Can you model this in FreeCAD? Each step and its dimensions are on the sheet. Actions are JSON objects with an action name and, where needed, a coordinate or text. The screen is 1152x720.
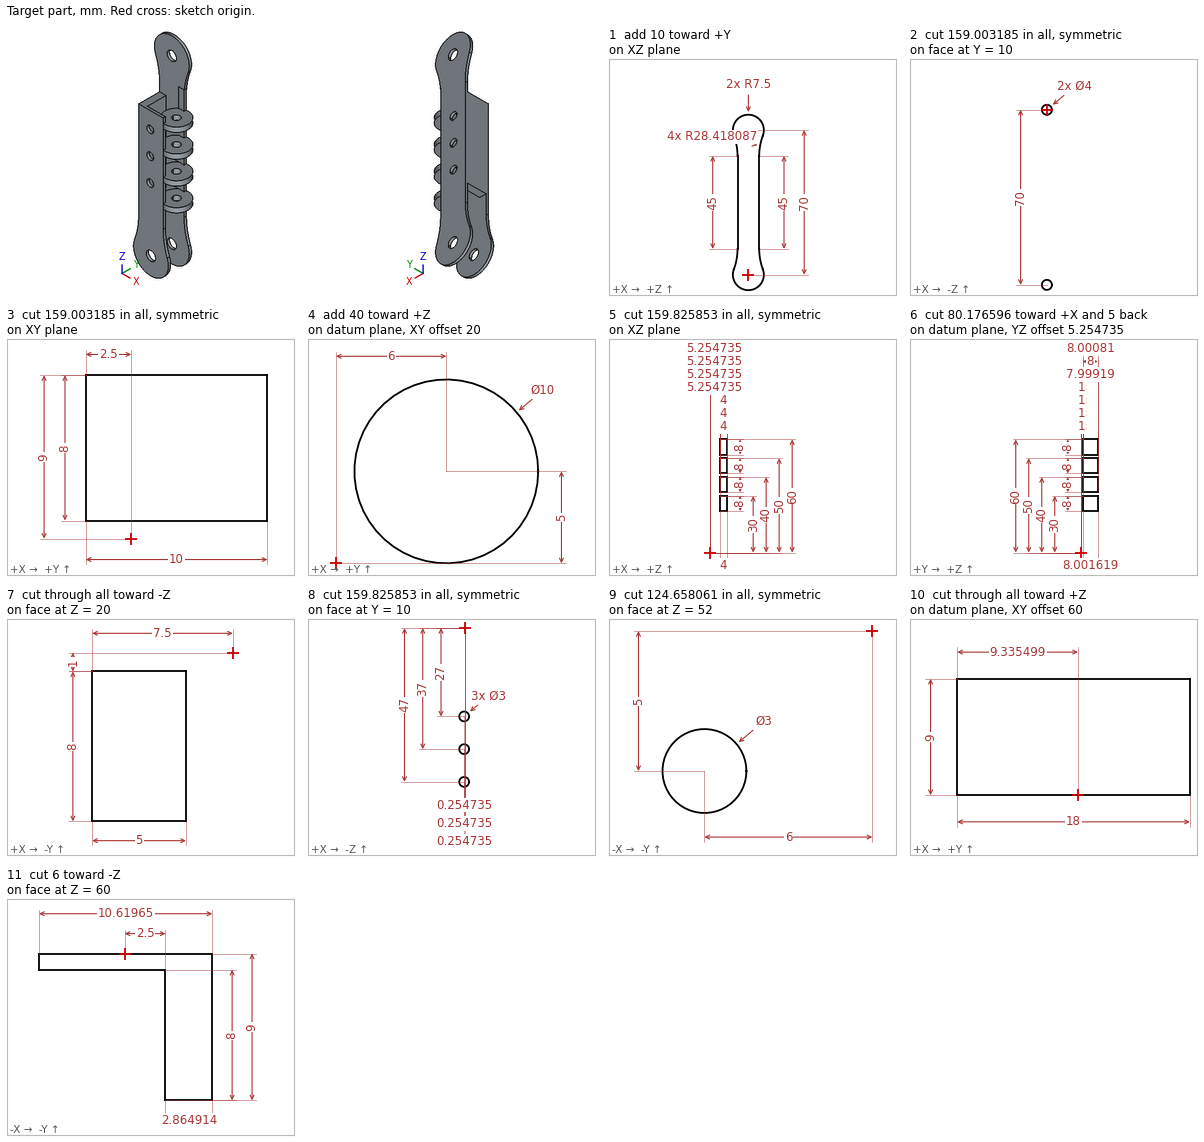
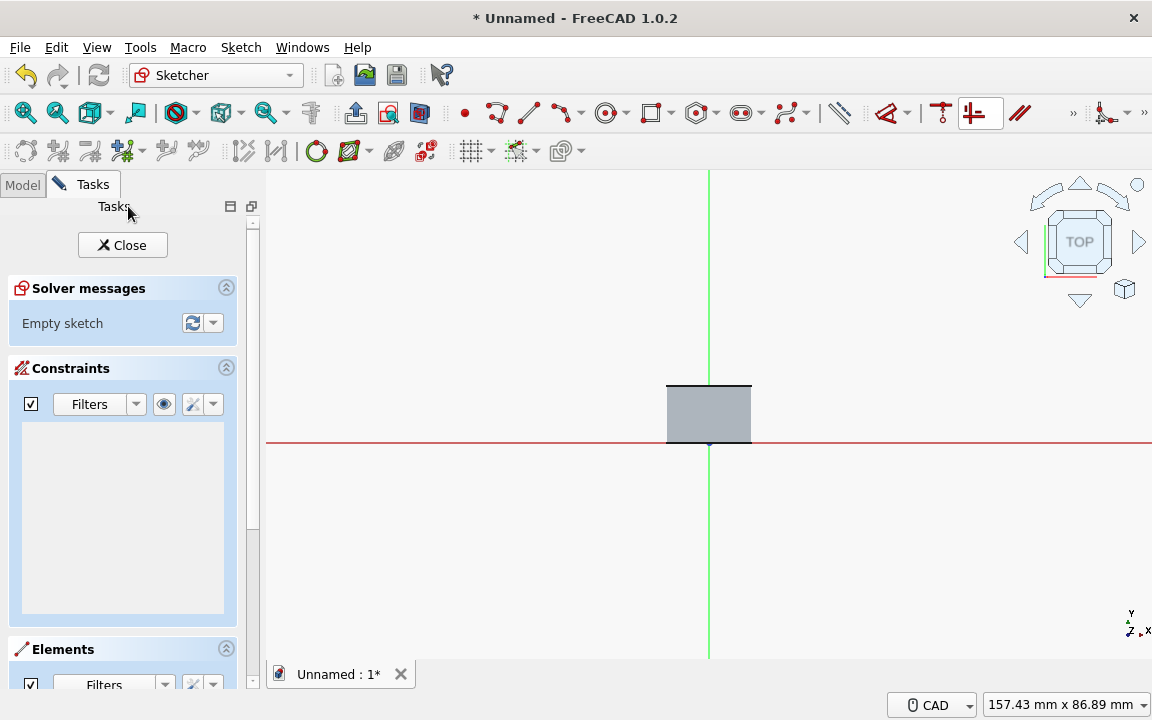
{"action": "left_click", "coordinate": [420, 114]}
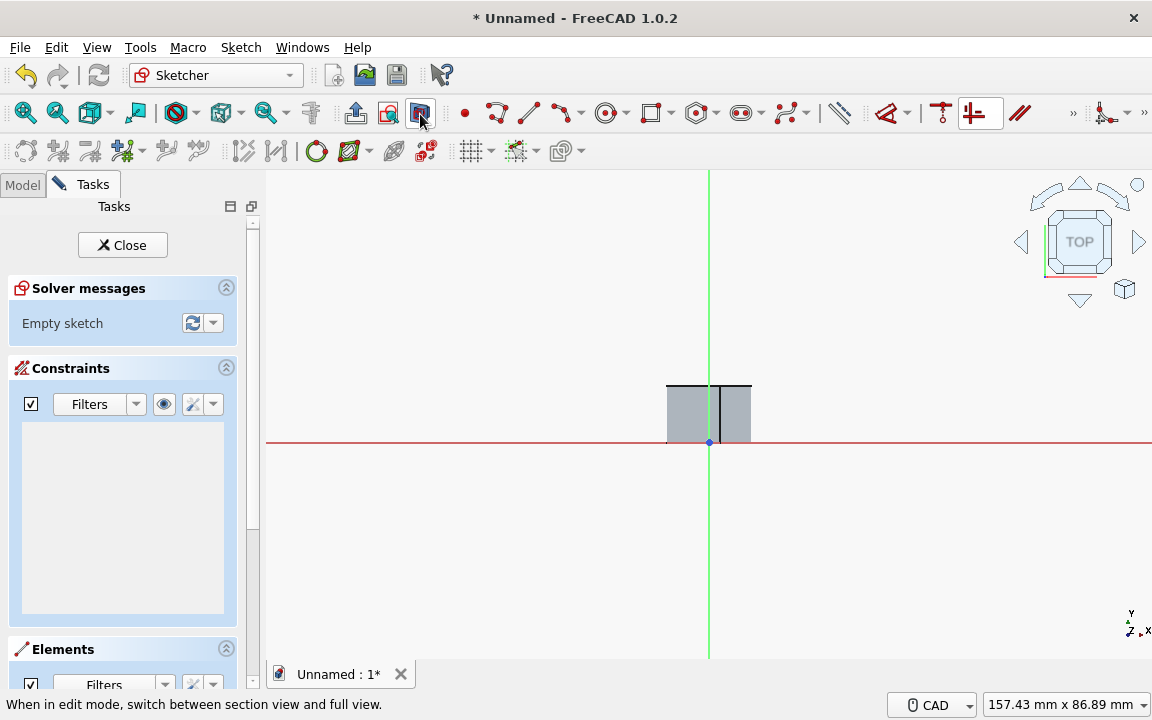
{"action": "scroll", "coordinate": [739, 418], "scroll_direction": "up", "scroll_amount": 9}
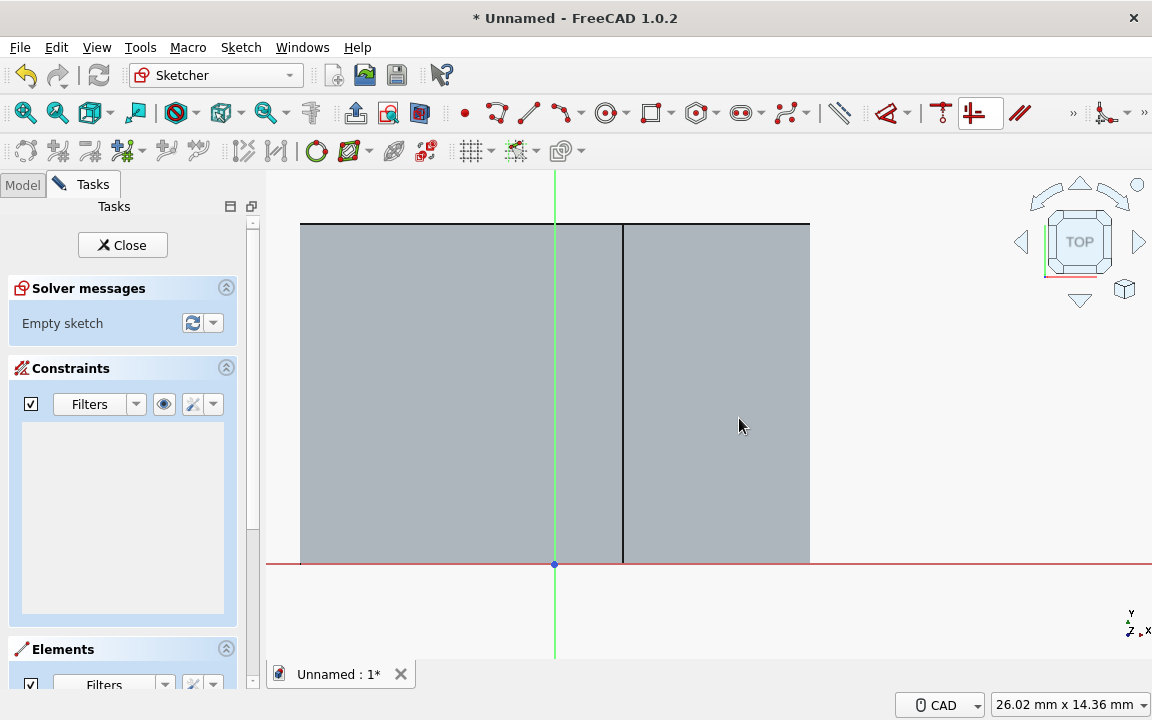
{"action": "left_click", "coordinate": [652, 114]}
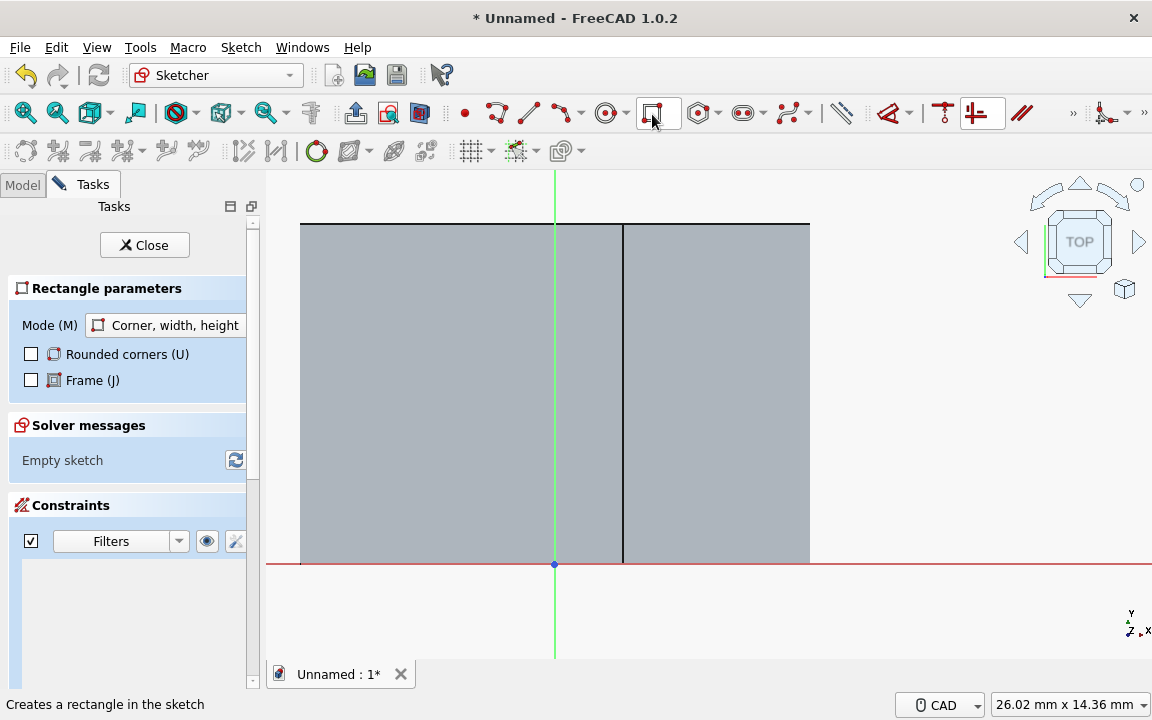
{"action": "left_click", "coordinate": [470, 258]}
{"action": "left_click", "coordinate": [810, 530]}
{"action": "key", "text": "Escape"}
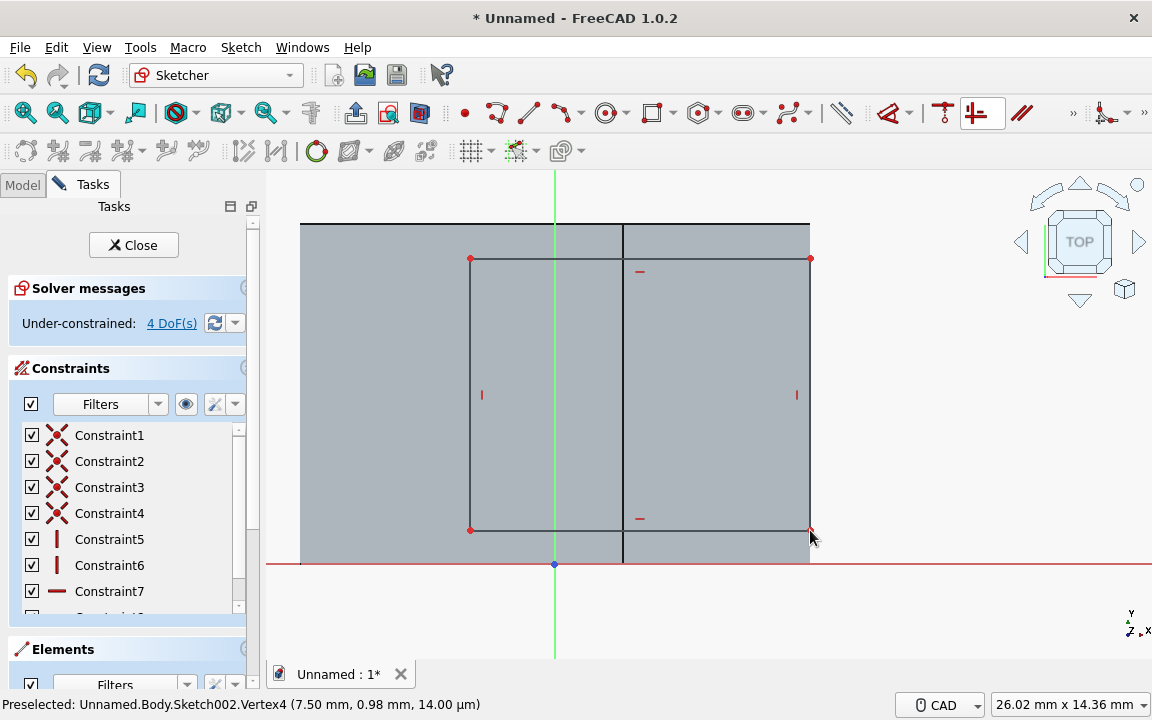
{"action": "key", "text": "d"}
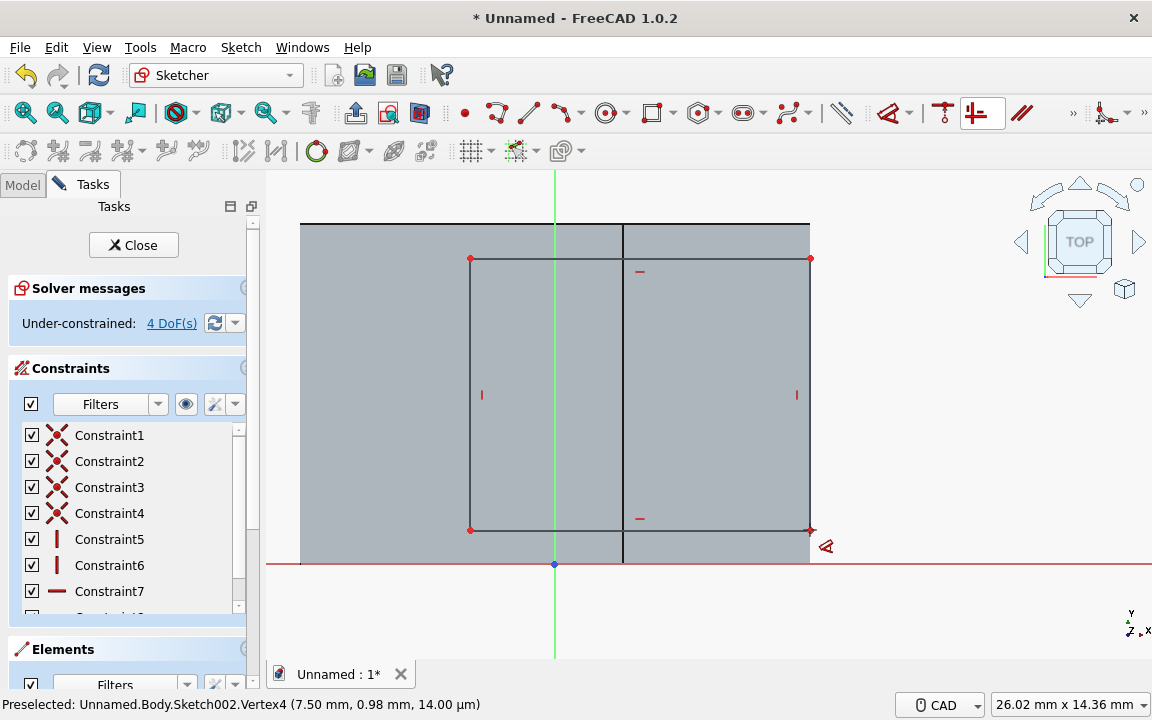
{"action": "left_click", "coordinate": [470, 341]}
{"action": "left_click", "coordinate": [436, 395]}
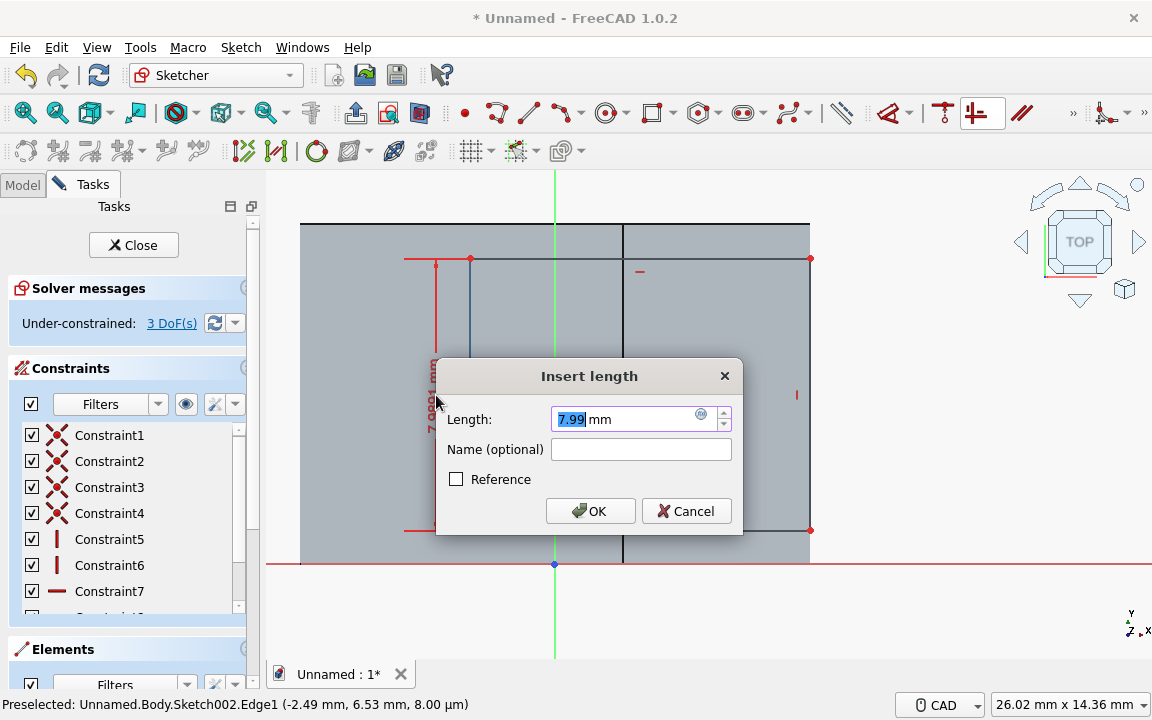
{"action": "type", "text": "8"}
{"action": "key", "text": "Return"}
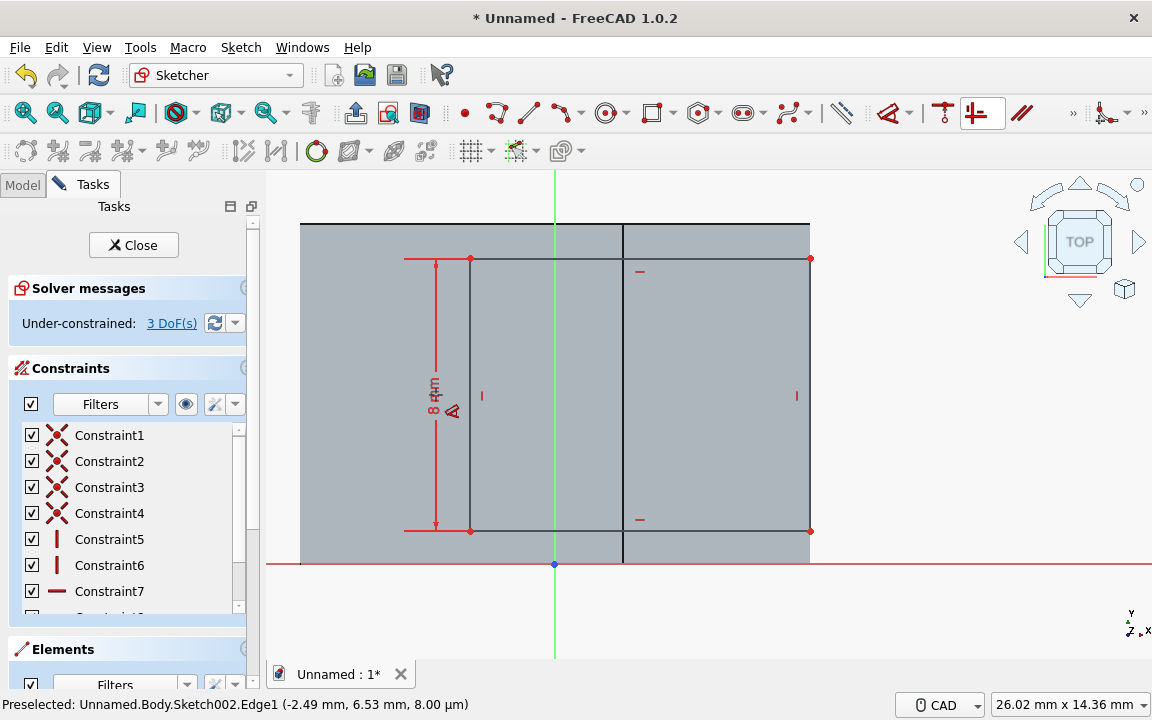
{"action": "left_click", "coordinate": [572, 531]}
{"action": "left_click", "coordinate": [640, 497]}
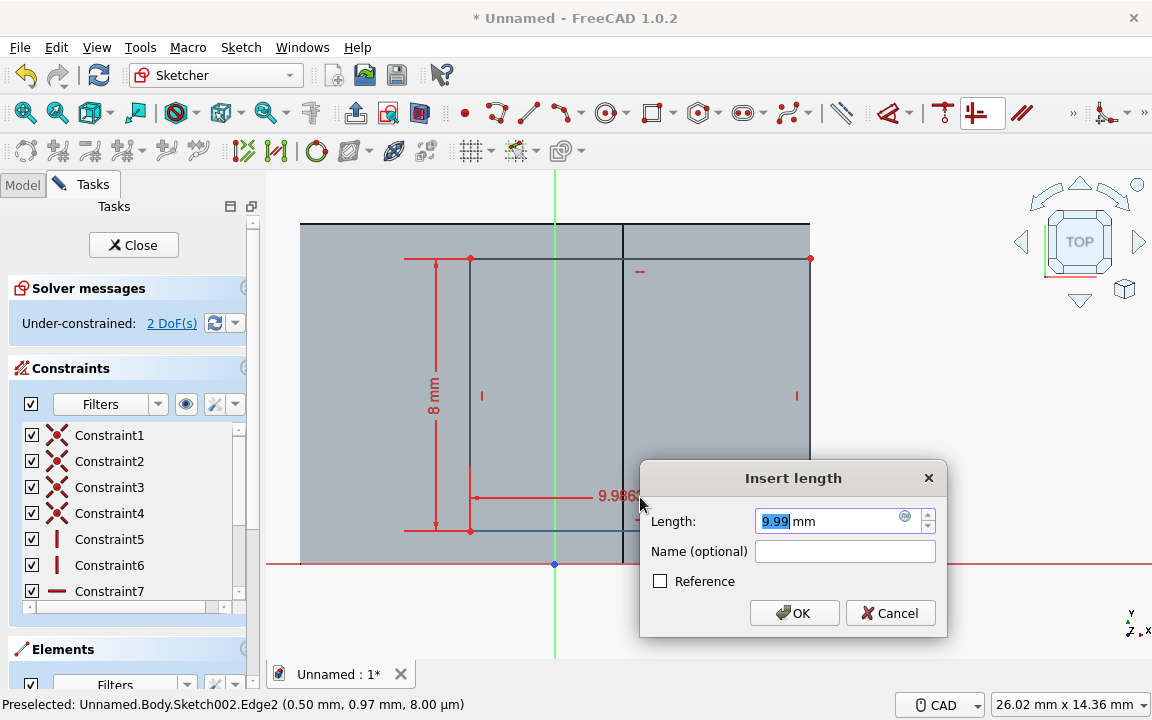
{"action": "type", "text": "10"}
{"action": "key", "text": "Return"}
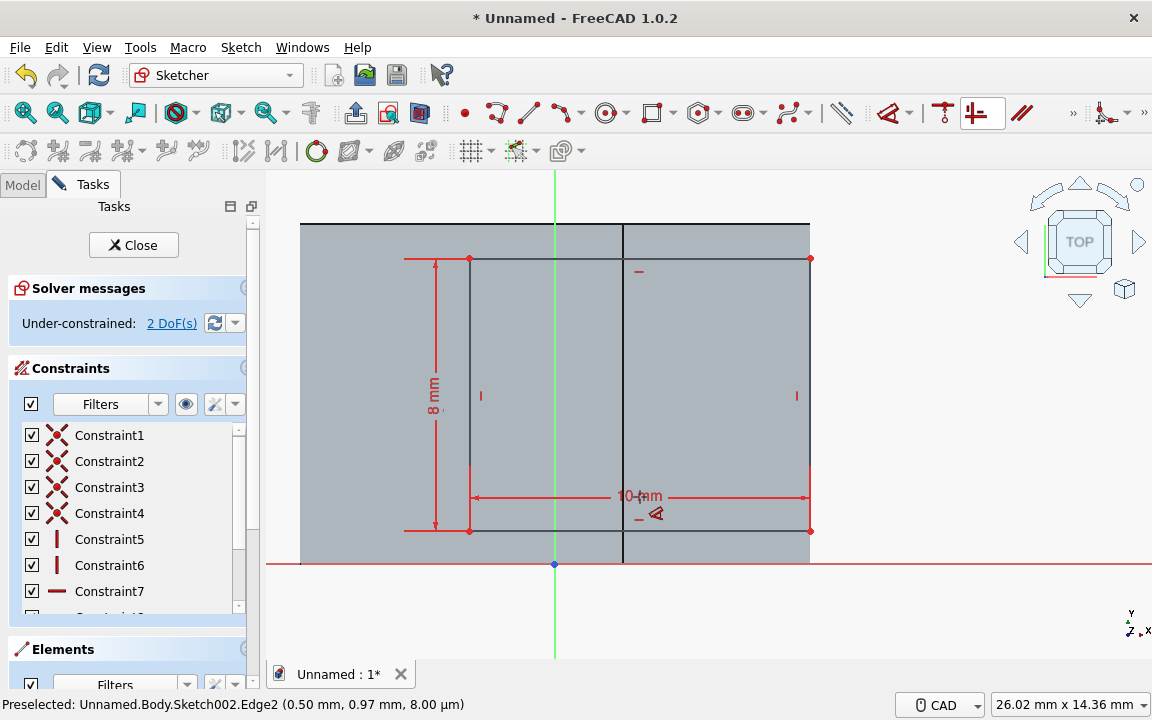
{"action": "left_click", "coordinate": [470, 259]}
{"action": "left_click", "coordinate": [436, 341]}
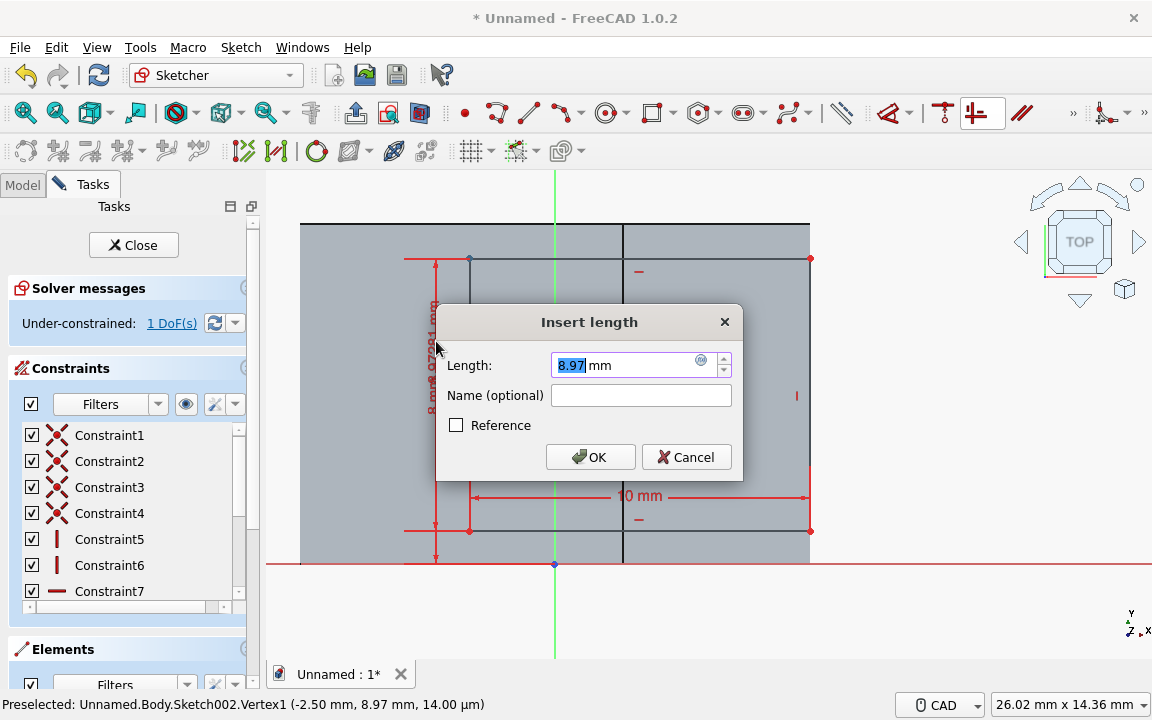
{"action": "type", "text": "9"}
{"action": "key", "text": "Return"}